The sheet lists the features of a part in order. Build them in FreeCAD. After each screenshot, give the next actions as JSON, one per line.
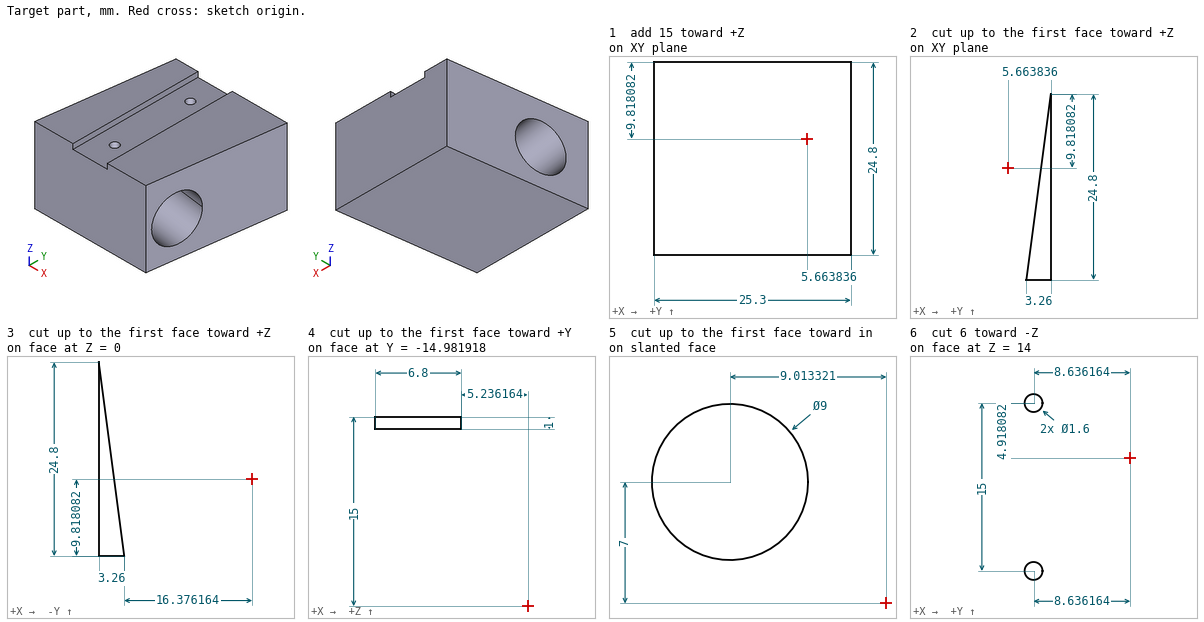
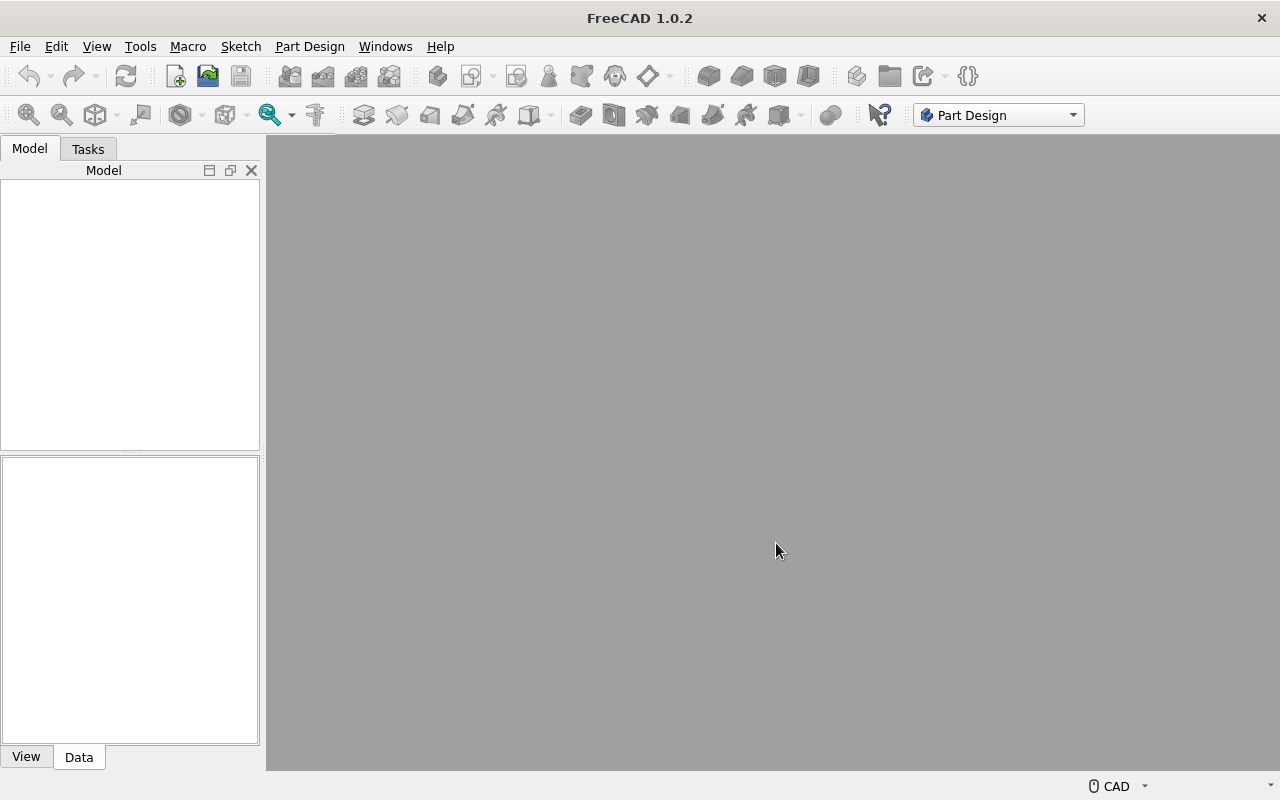
{"action": "key", "text": "ctrl+n"}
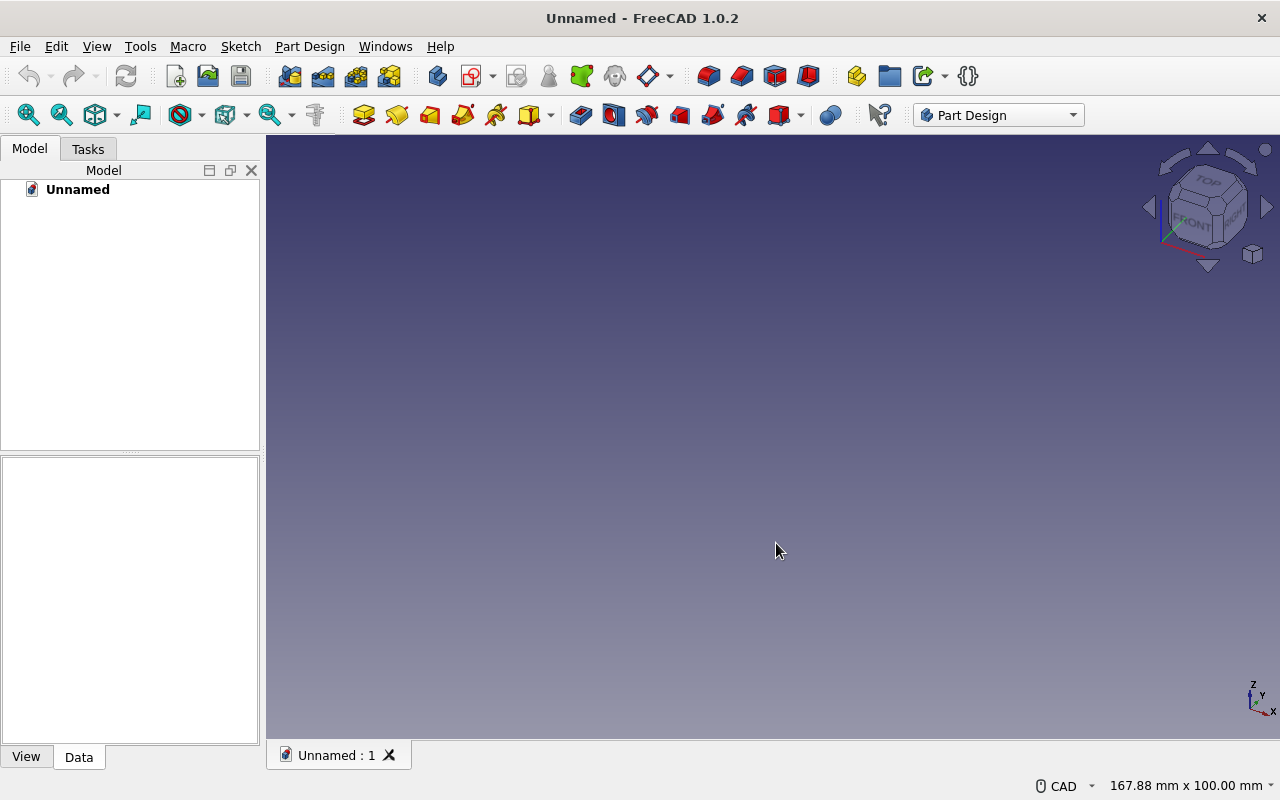
{"action": "left_click", "coordinate": [470, 76]}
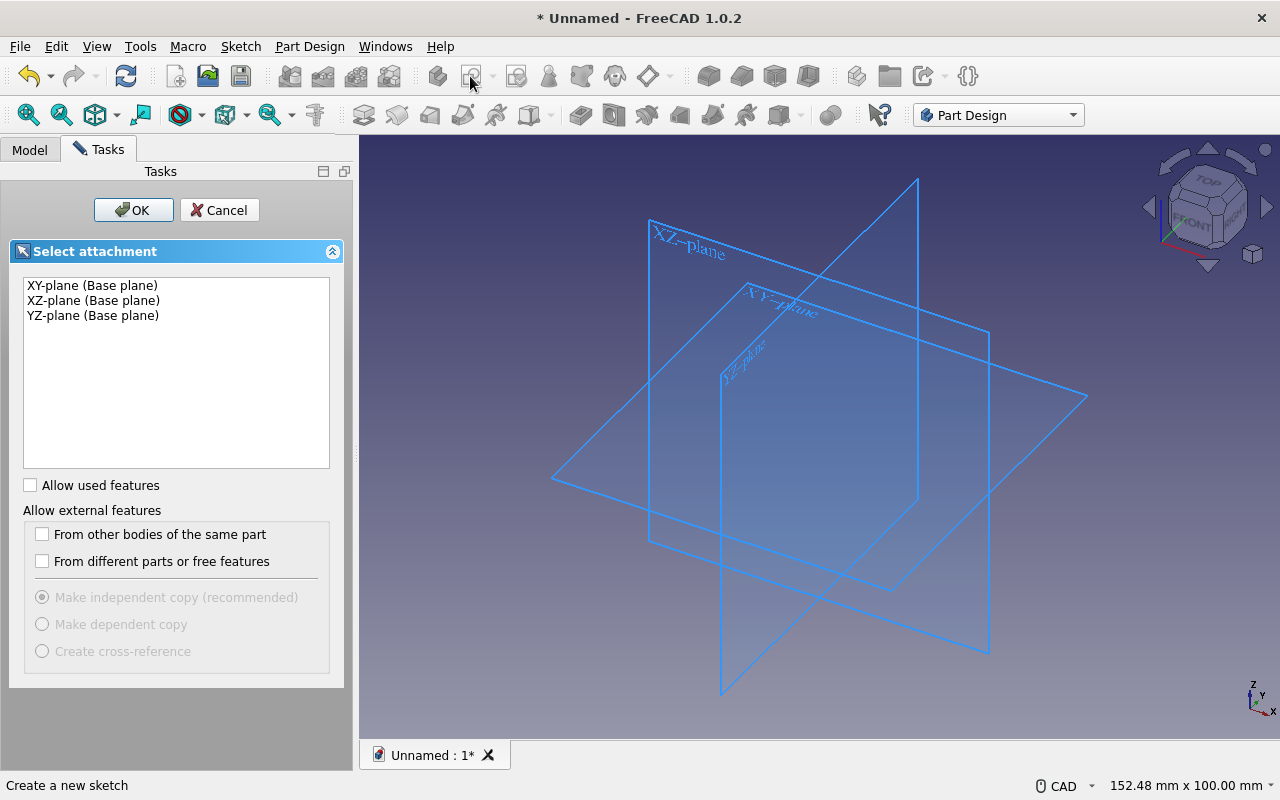
{"action": "left_click", "coordinate": [84, 286]}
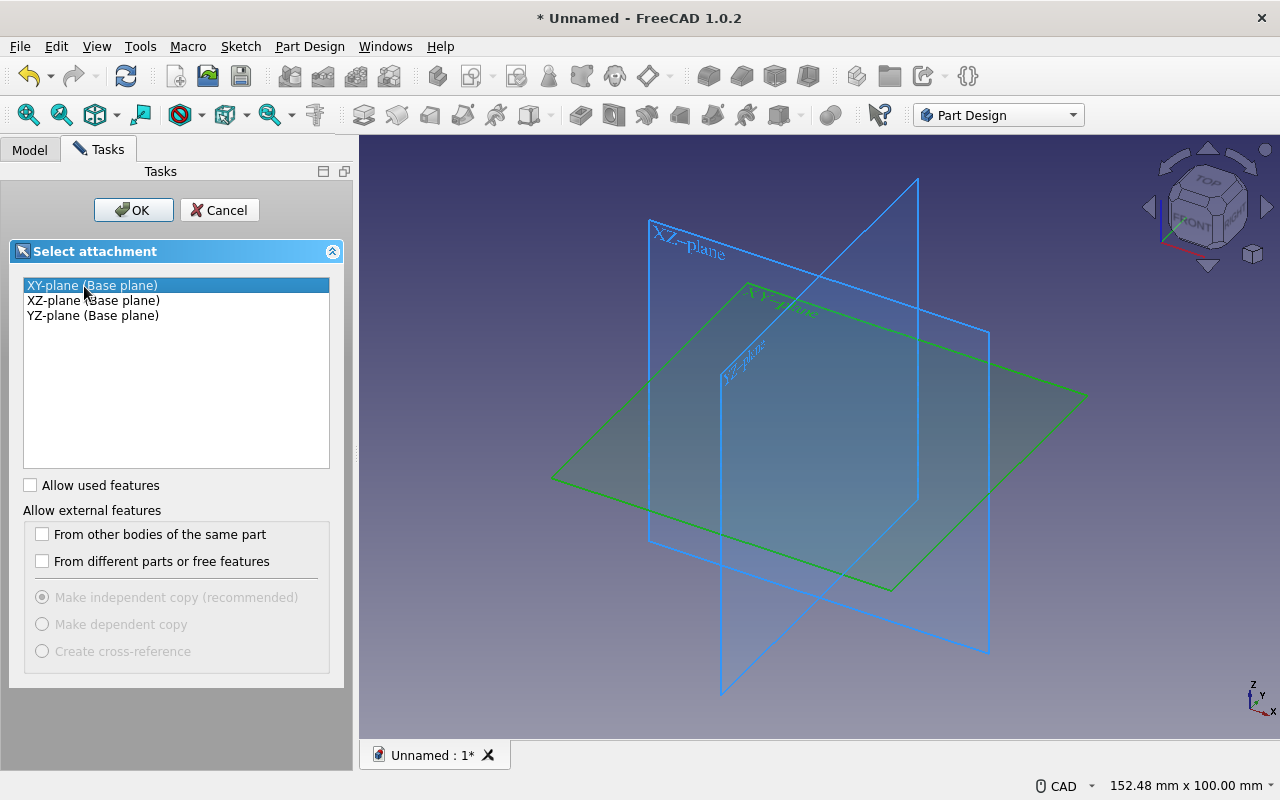
{"action": "left_click", "coordinate": [134, 210]}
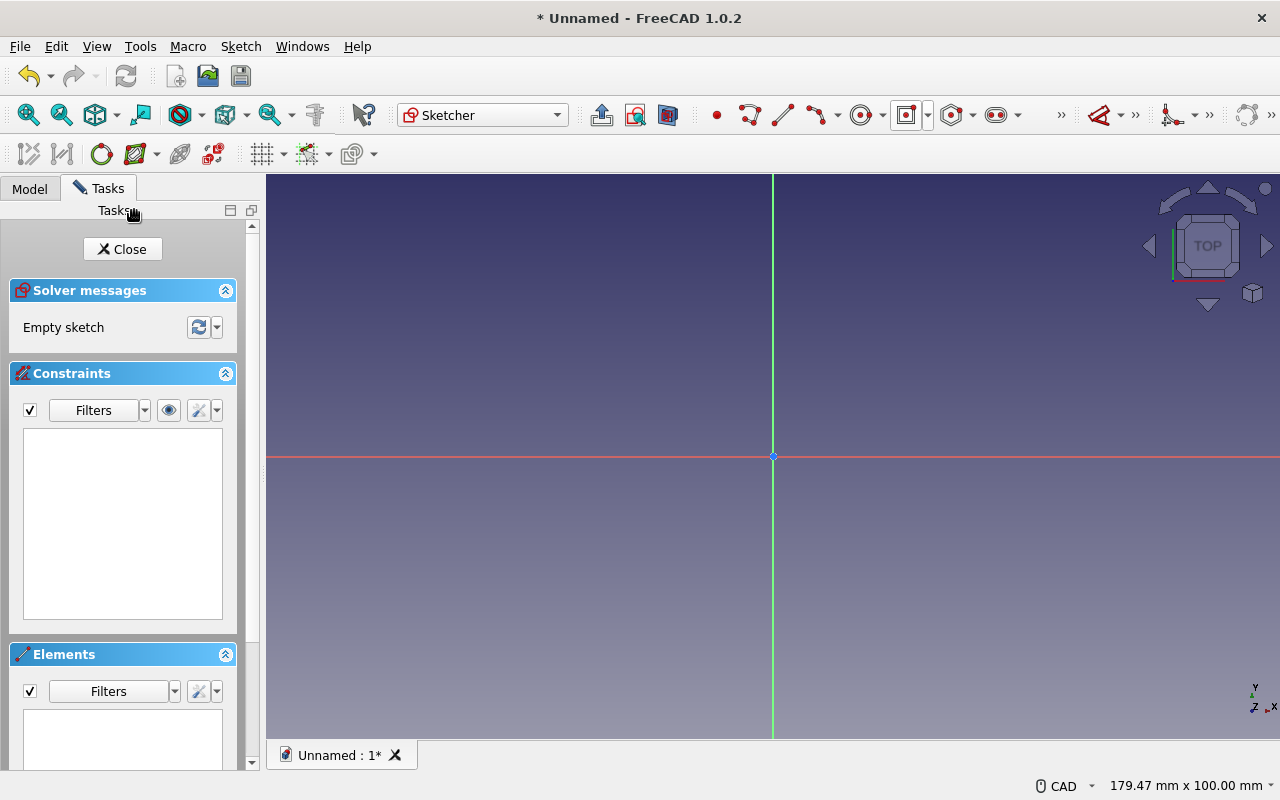
{"action": "scroll", "coordinate": [750, 480], "scroll_direction": "up", "scroll_amount": 5}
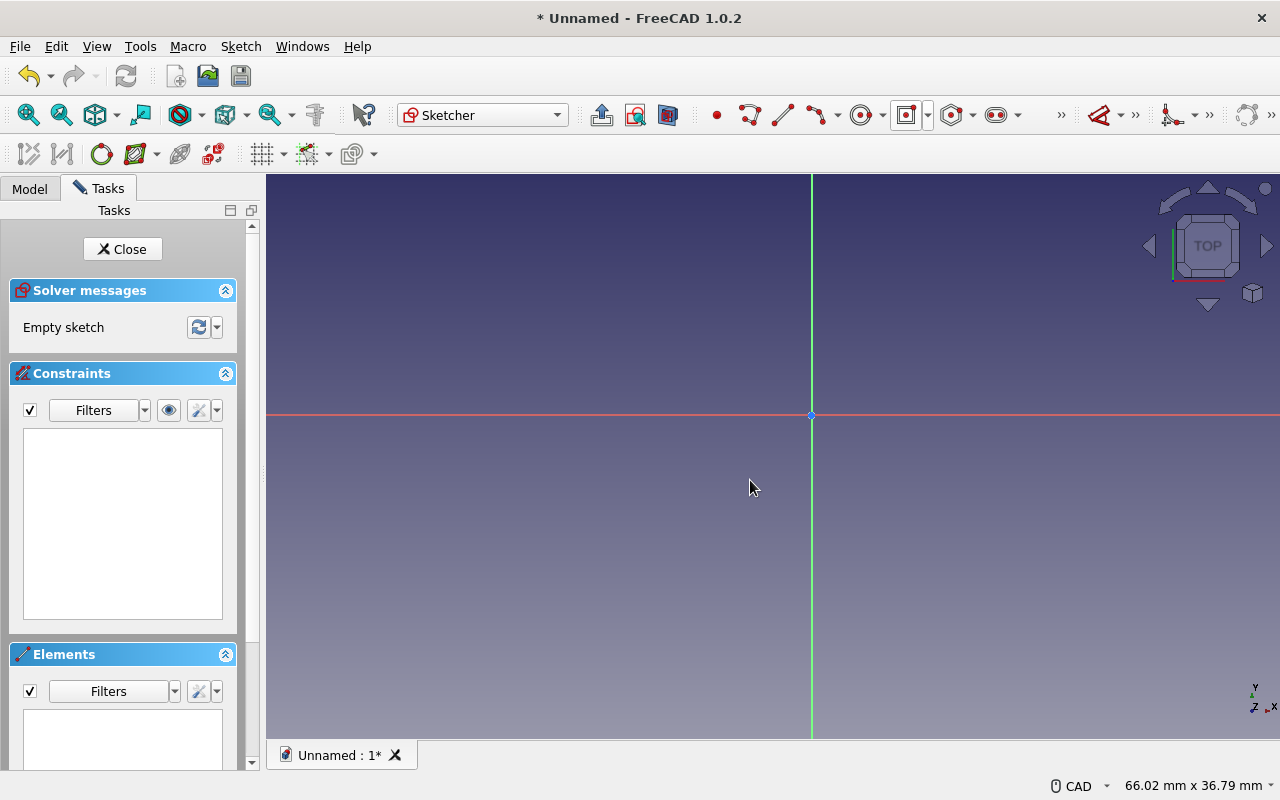
{"action": "left_click", "coordinate": [928, 116]}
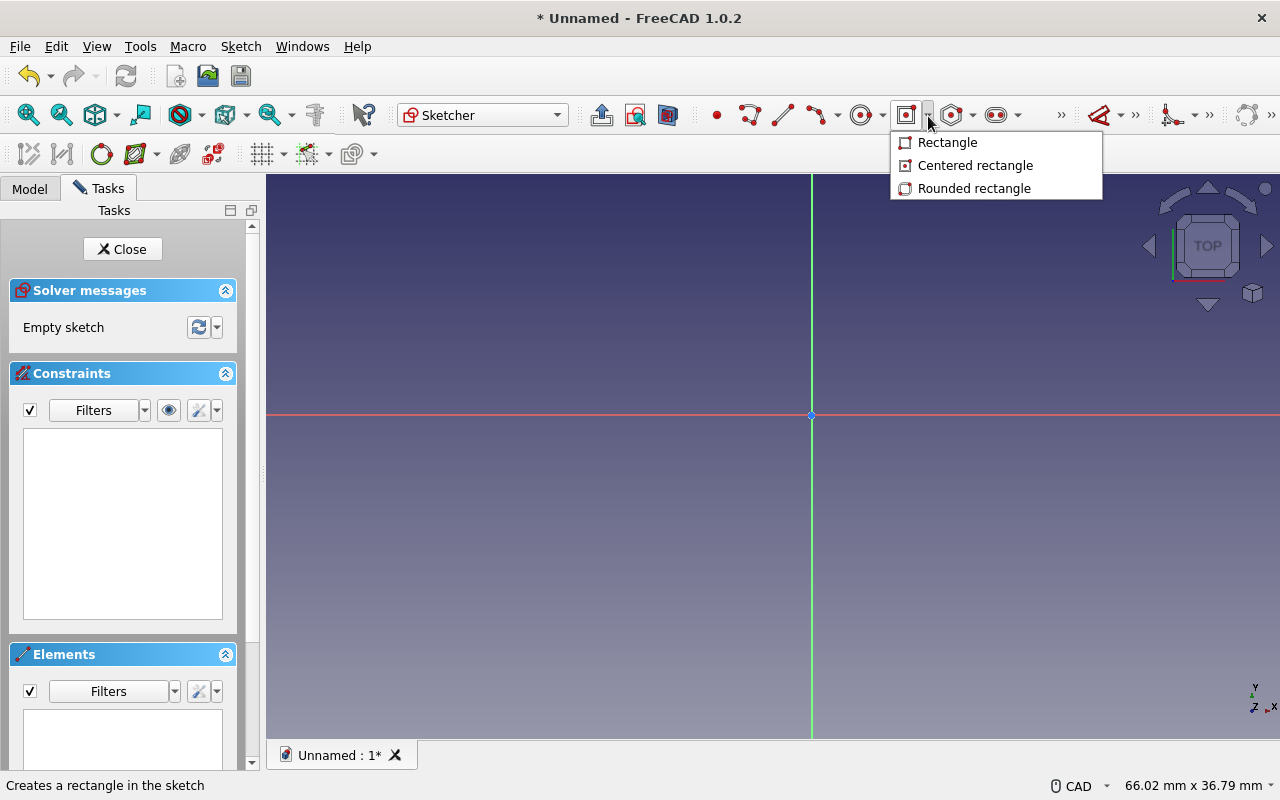
{"action": "left_click", "coordinate": [996, 142]}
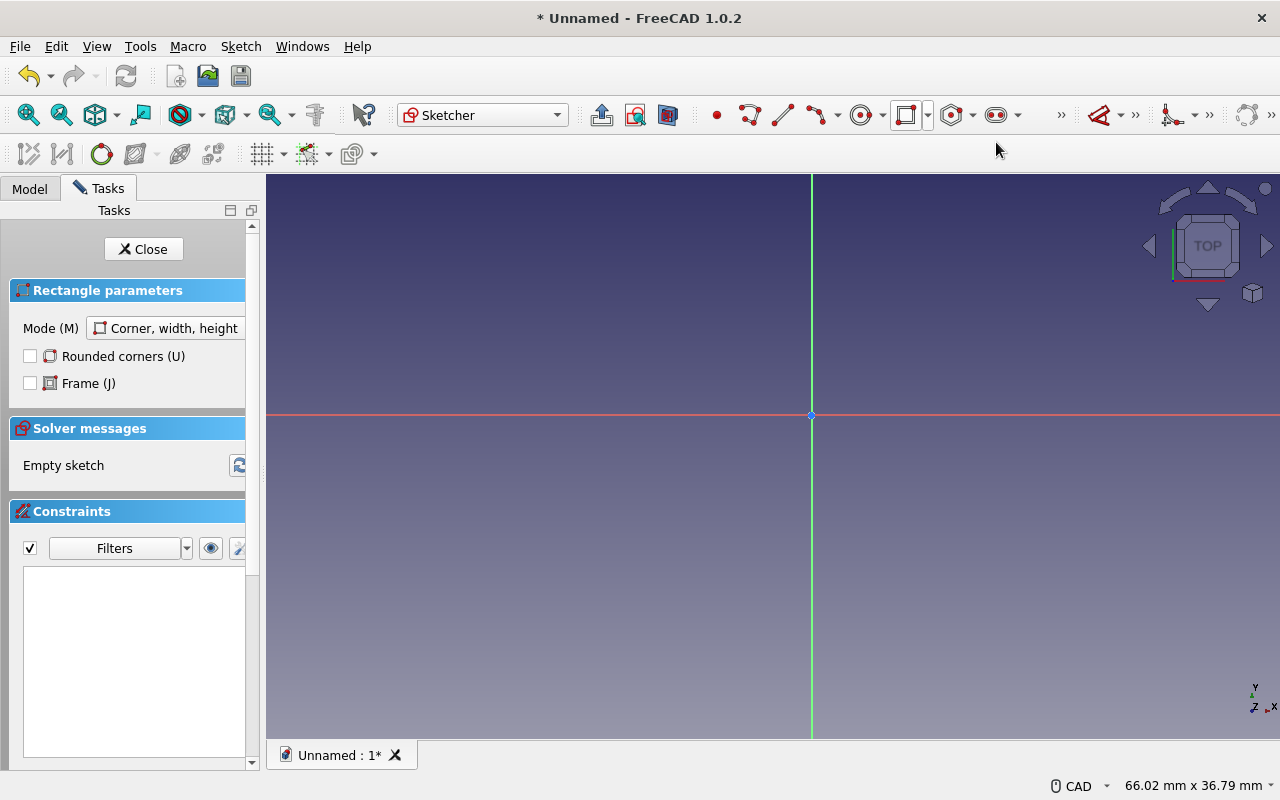
{"action": "left_click", "coordinate": [510, 264]}
{"action": "mouse_move", "coordinate": [899, 645]}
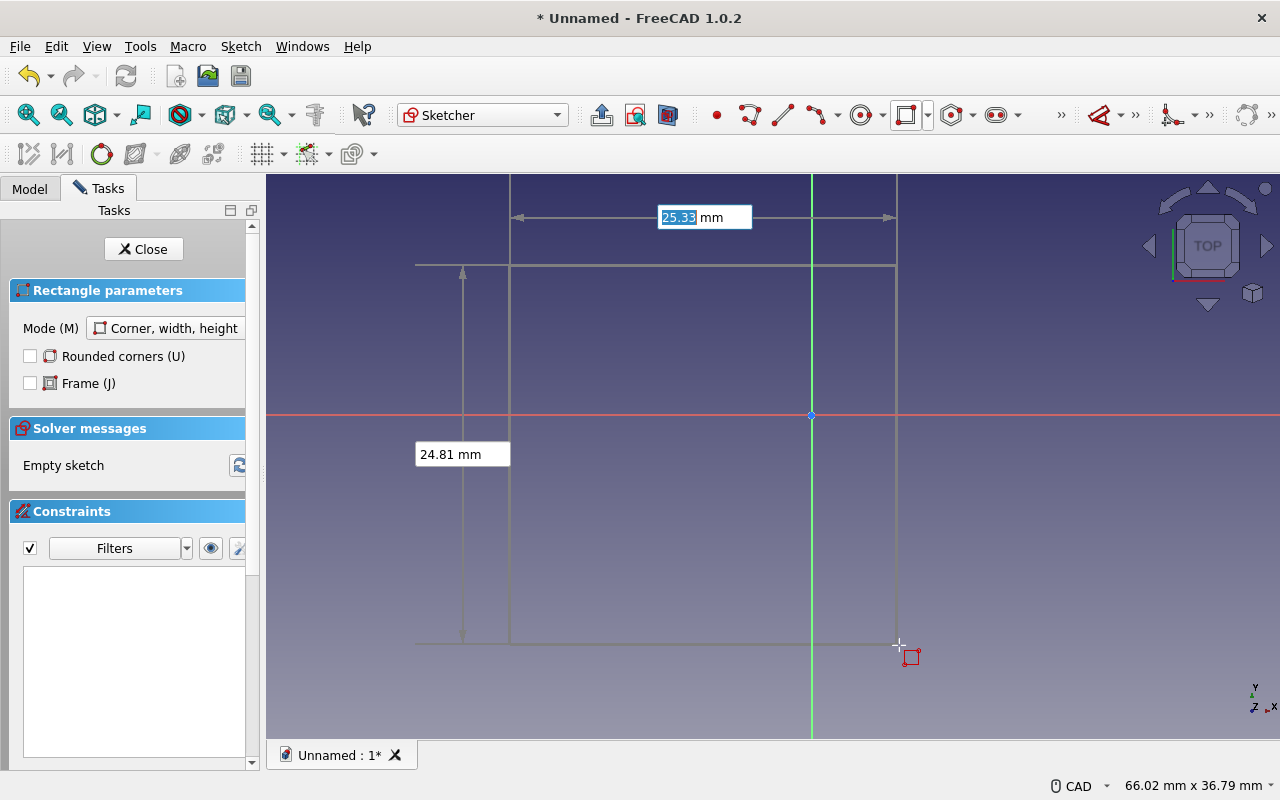
{"action": "type", "text": "25.3"}
{"action": "key", "text": "Tab"}
{"action": "type", "text": "24.8"}
{"action": "key", "text": "Return"}
{"action": "key", "text": "Escape"}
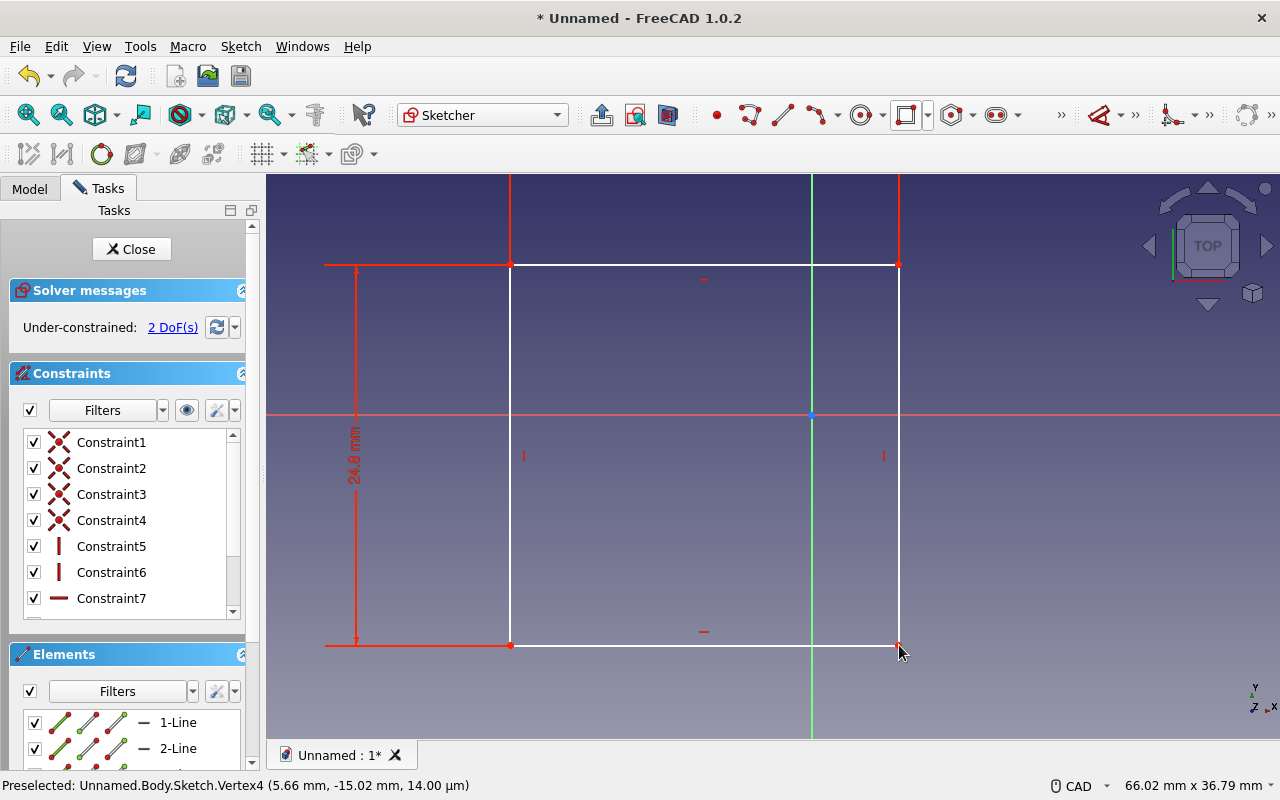
{"action": "left_click", "coordinate": [1098, 116]}